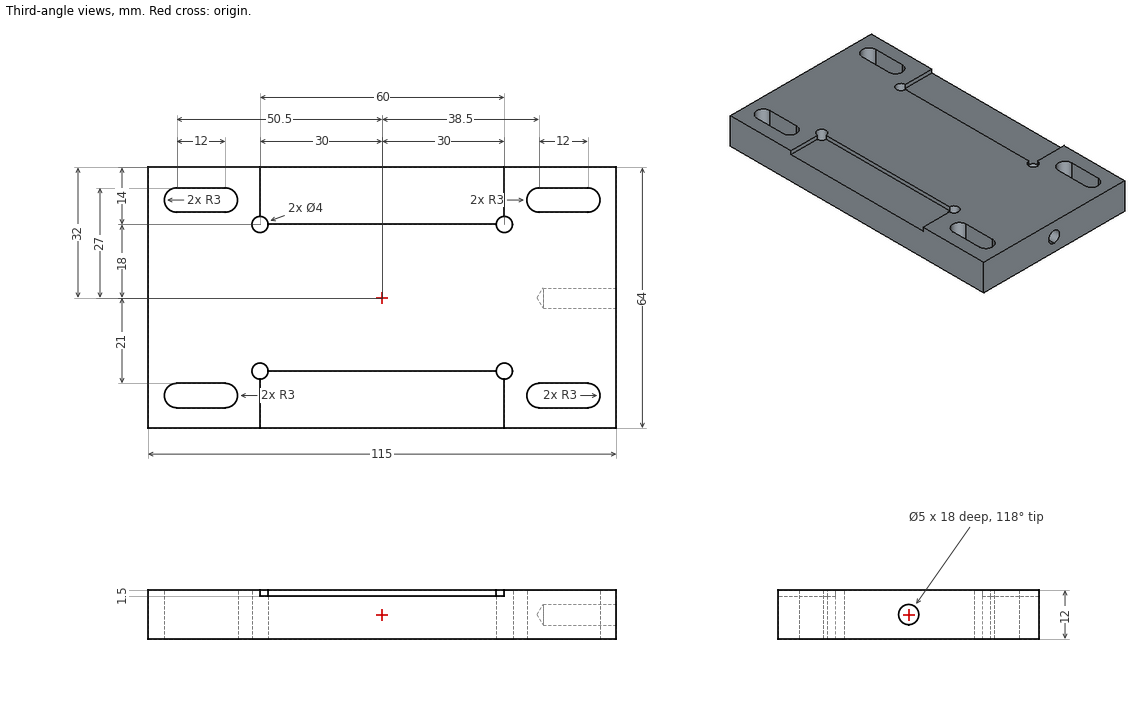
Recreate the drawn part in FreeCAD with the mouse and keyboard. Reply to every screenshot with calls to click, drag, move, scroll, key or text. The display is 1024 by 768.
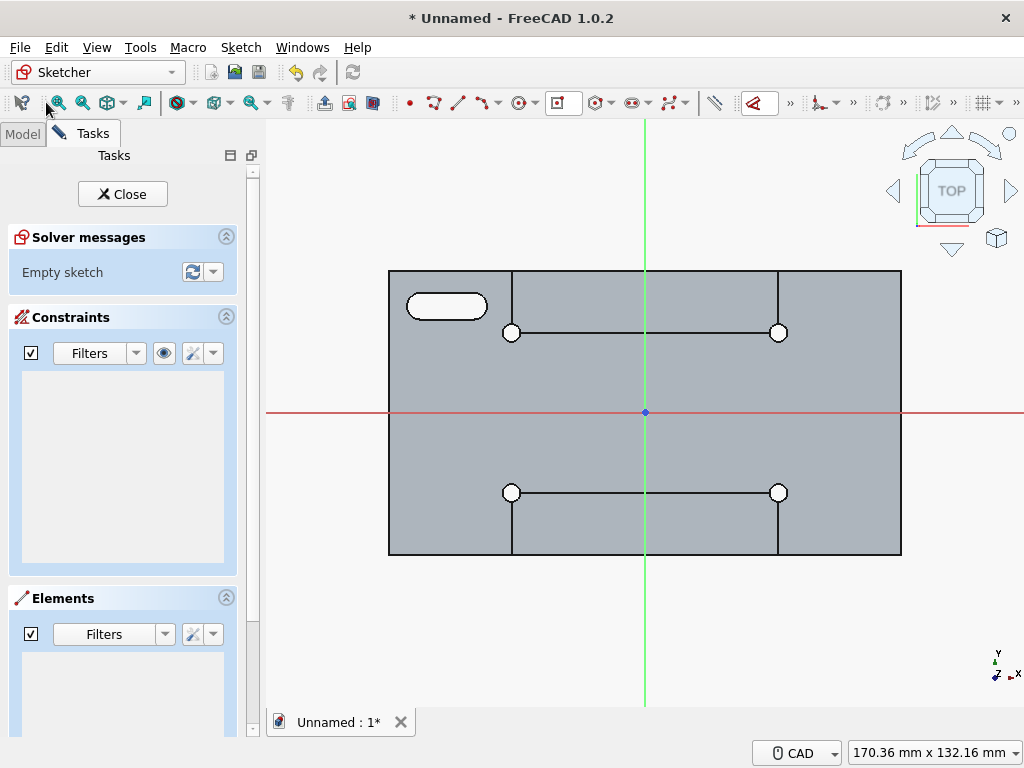
scroll(576, 413, down, 5)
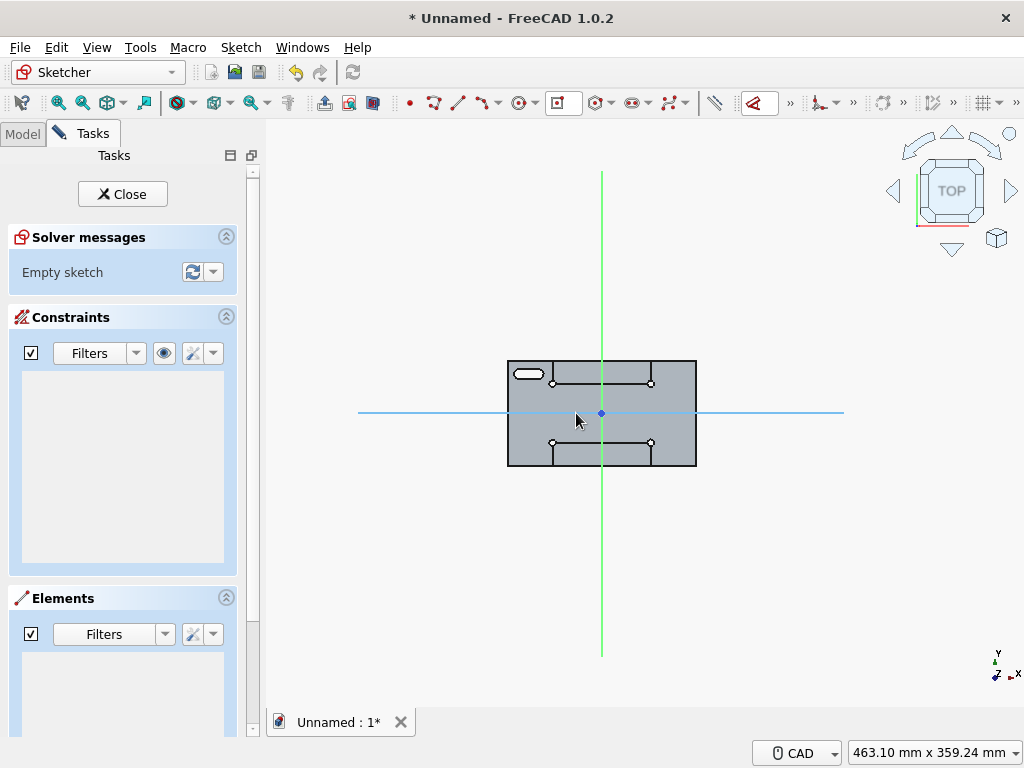
scroll(682, 371, up, 13)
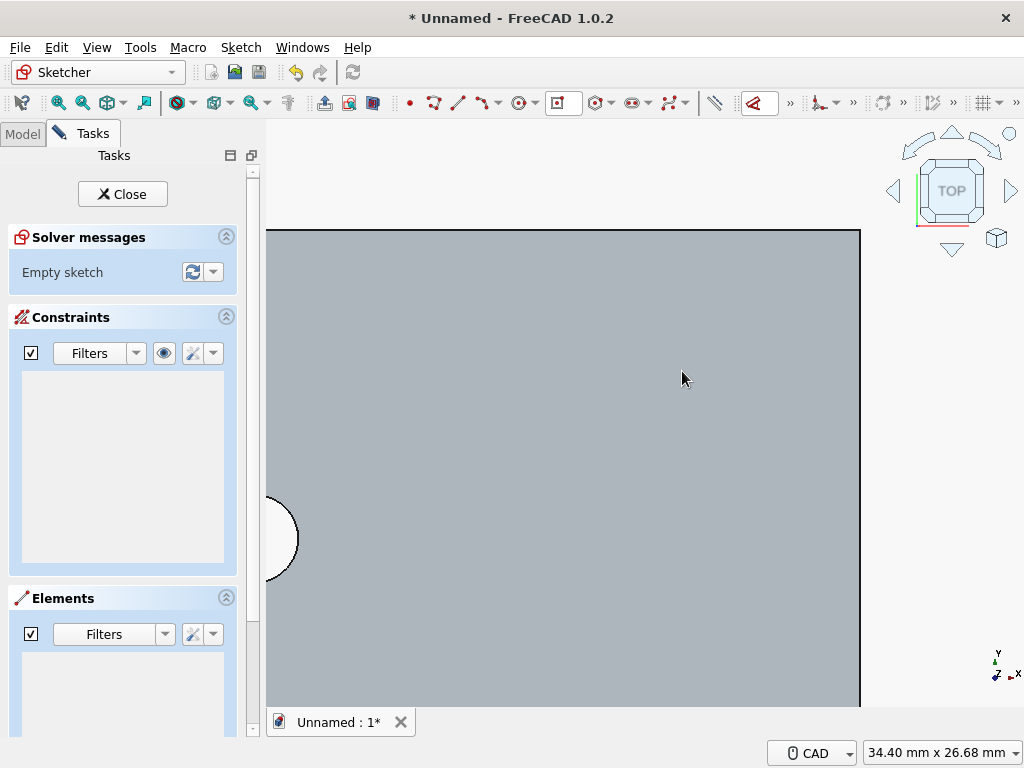
click(632, 104)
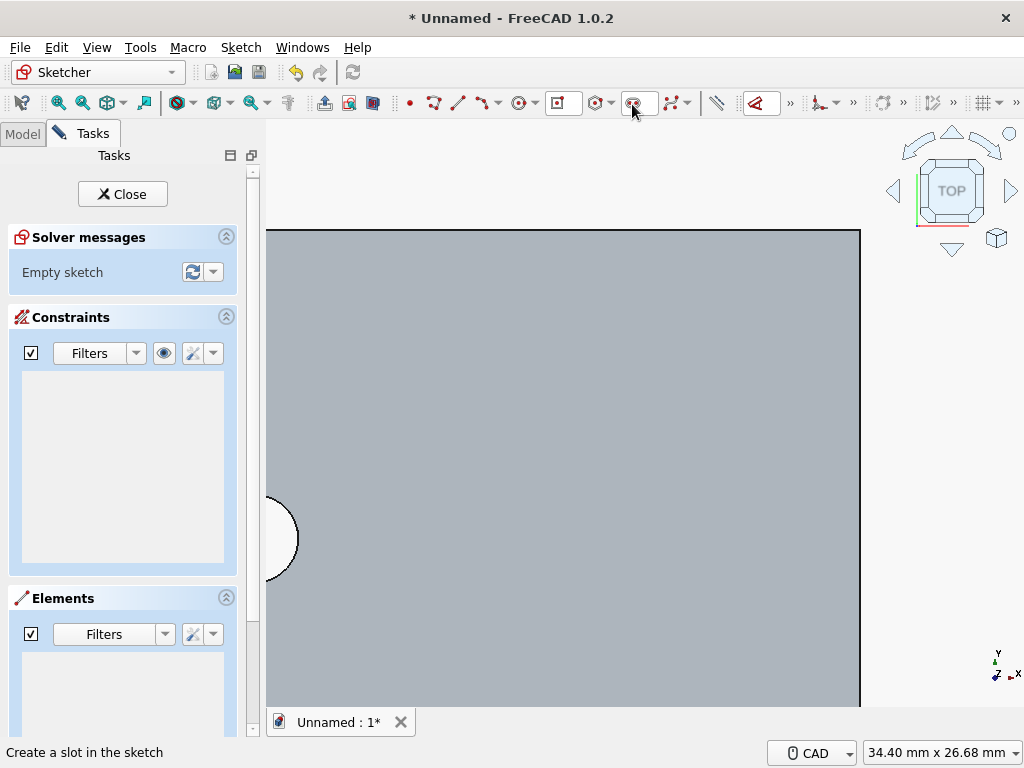
click(442, 406)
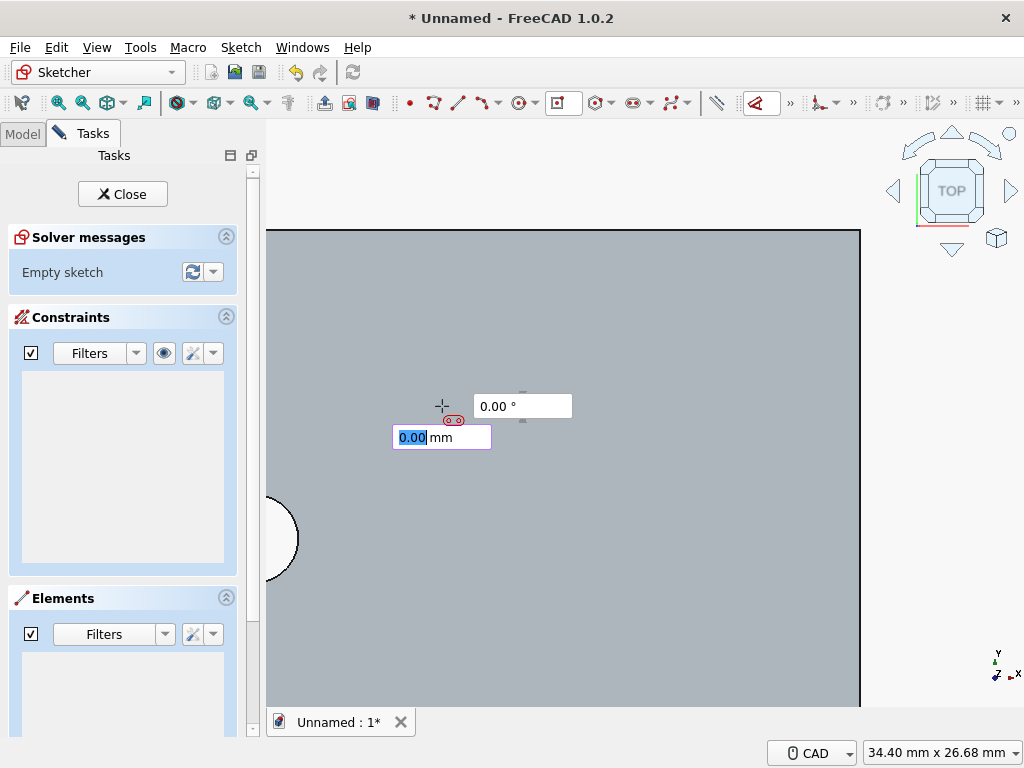
click(706, 406)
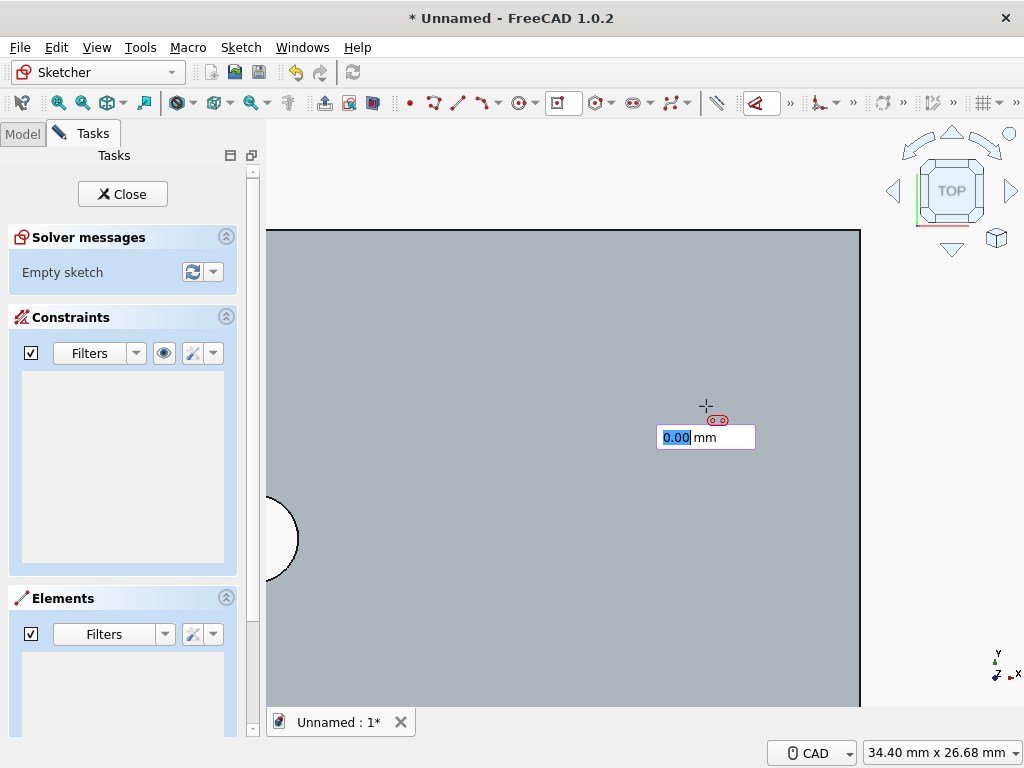
click(574, 340)
key(Escape)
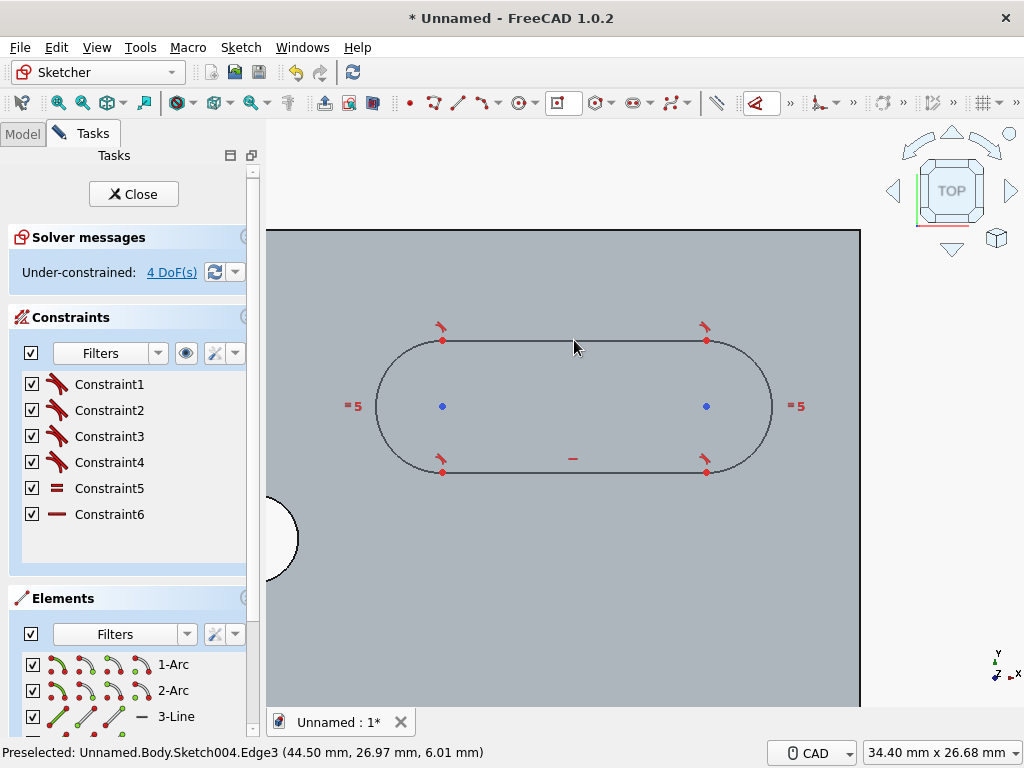
click(389, 368)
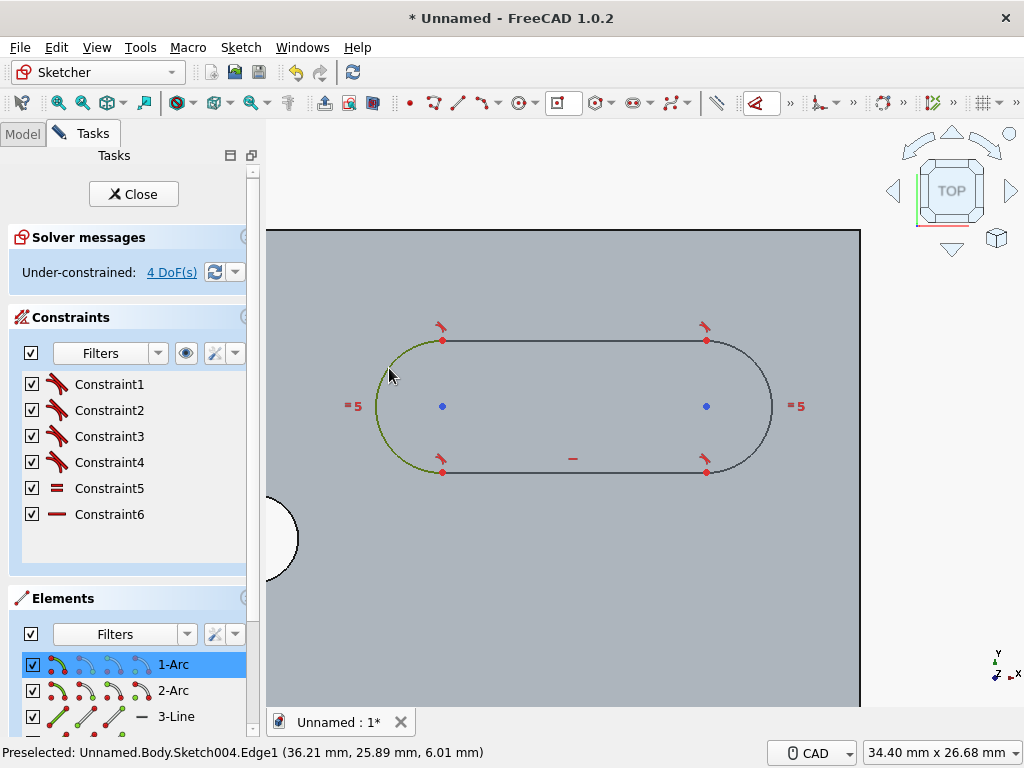
key(k)
key(r)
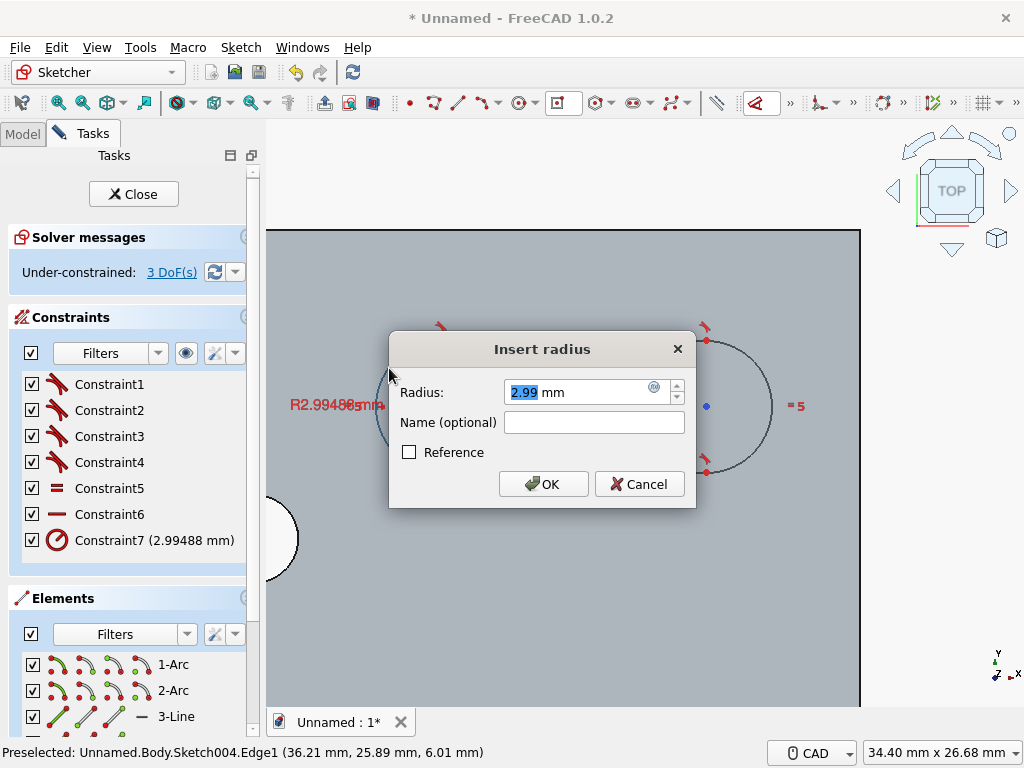
text(3)
key(Return)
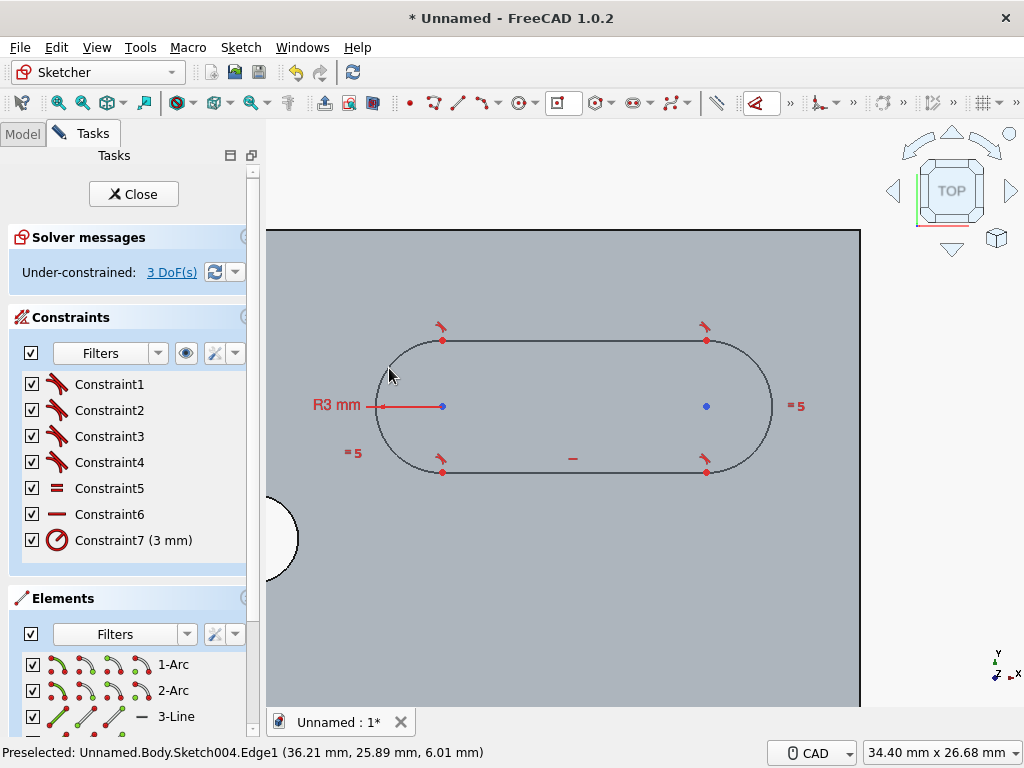
click(521, 341)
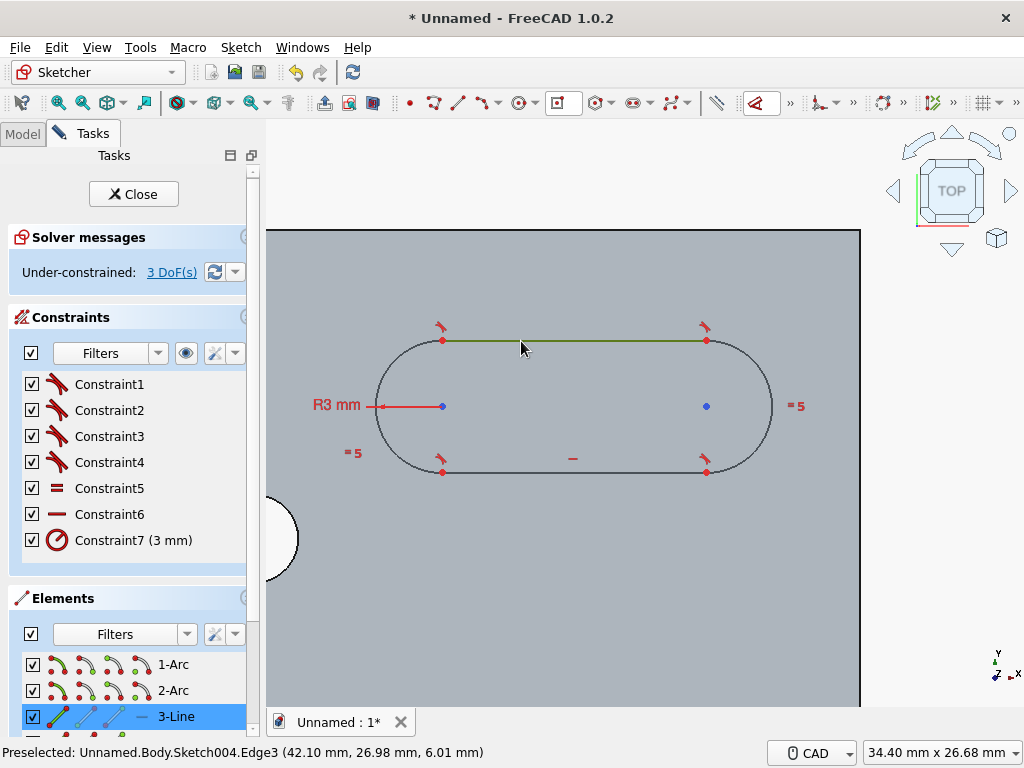
key(l)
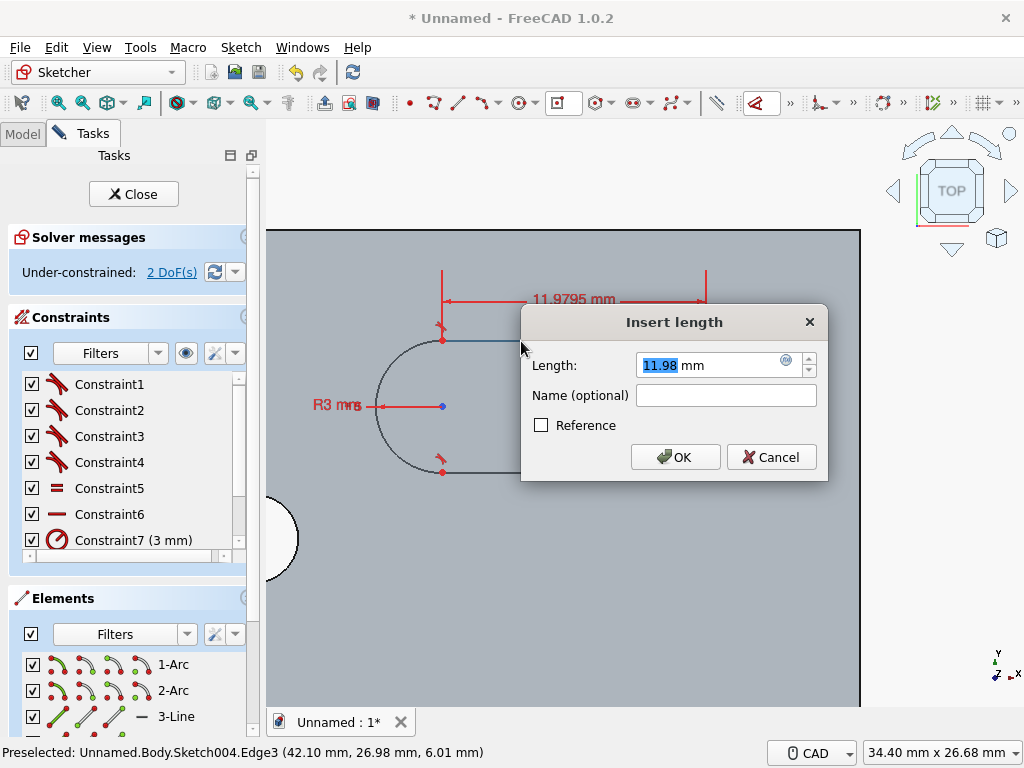
text(12)
key(Return)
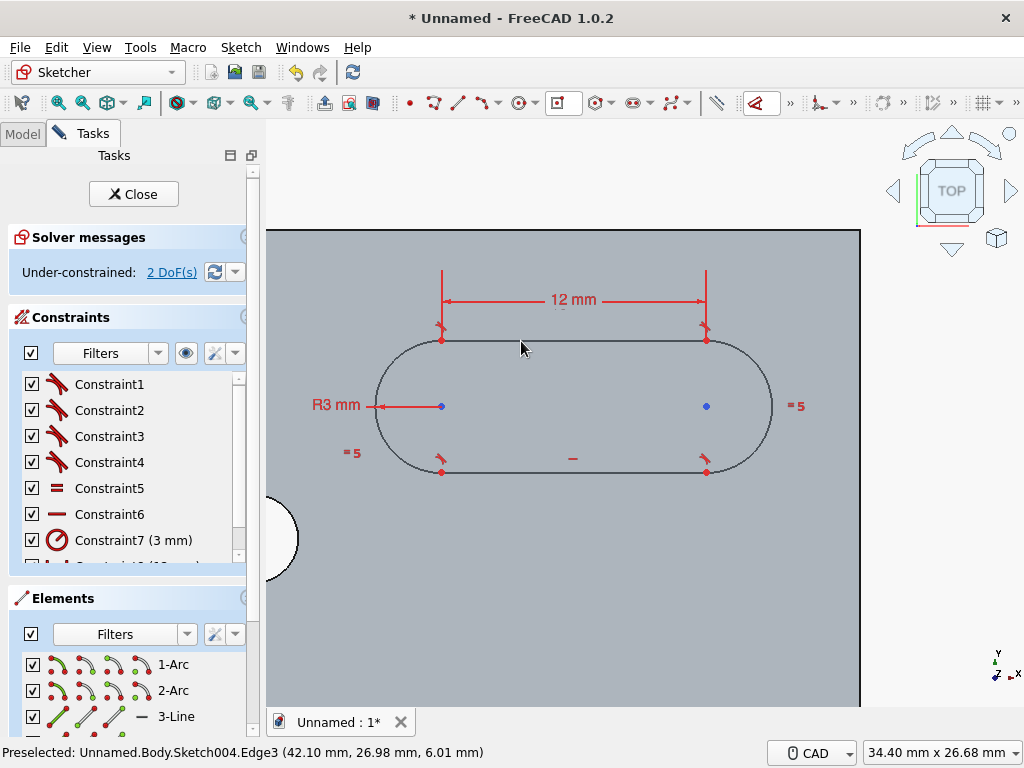
click(442, 341)